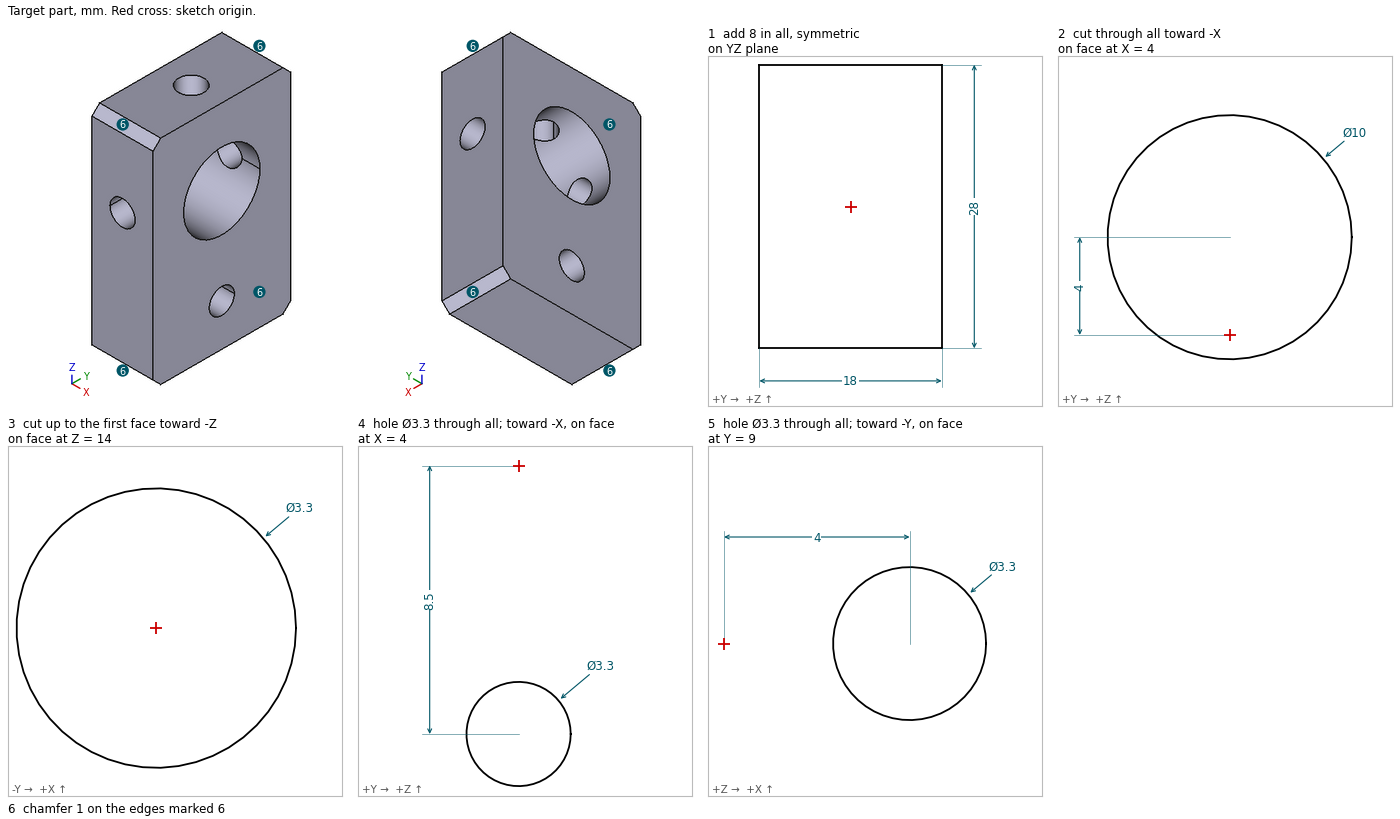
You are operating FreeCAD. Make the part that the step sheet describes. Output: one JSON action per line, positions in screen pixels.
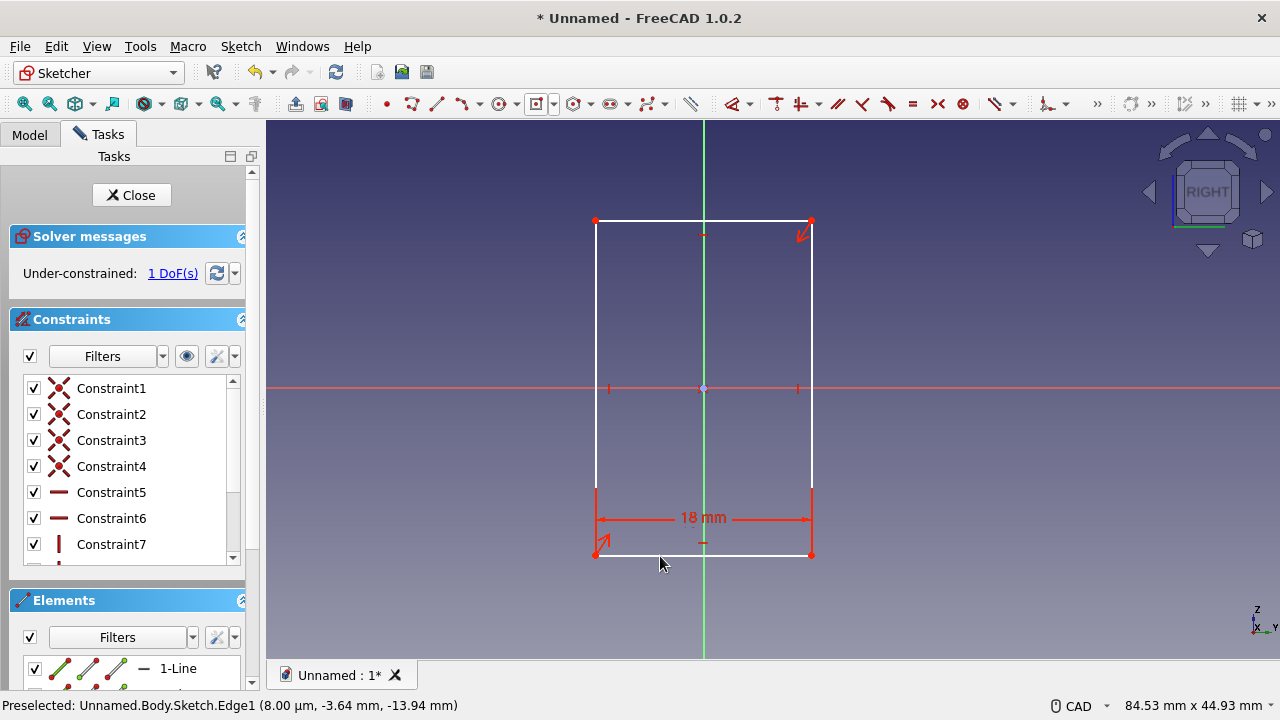
{"action": "left_click", "coordinate": [812, 455]}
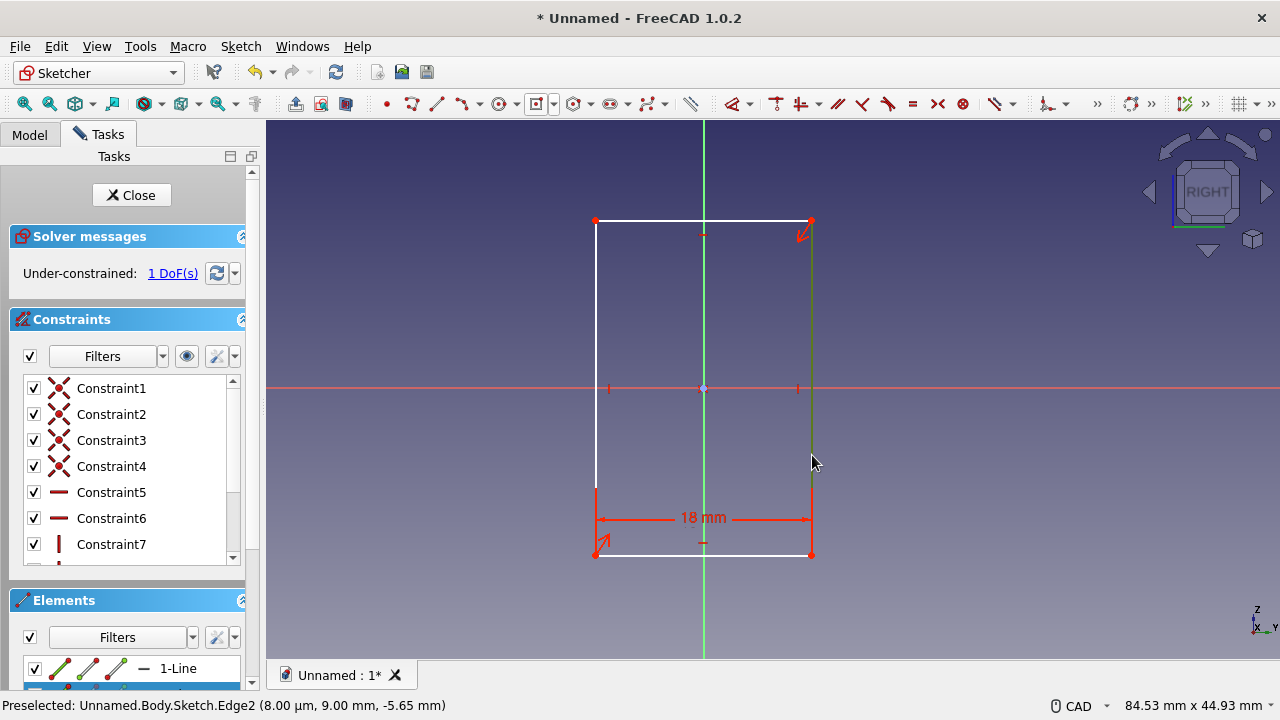
{"action": "key", "text": "i"}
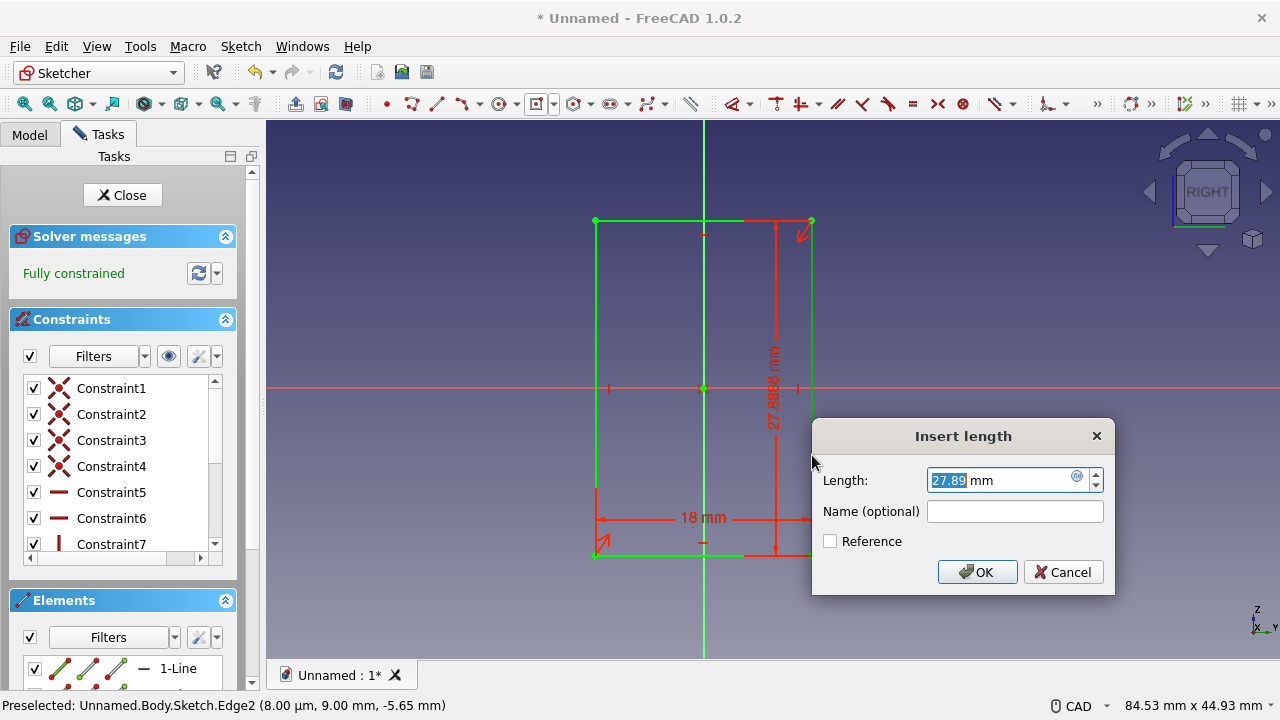
{"action": "type", "text": "28"}
{"action": "key", "text": "Return"}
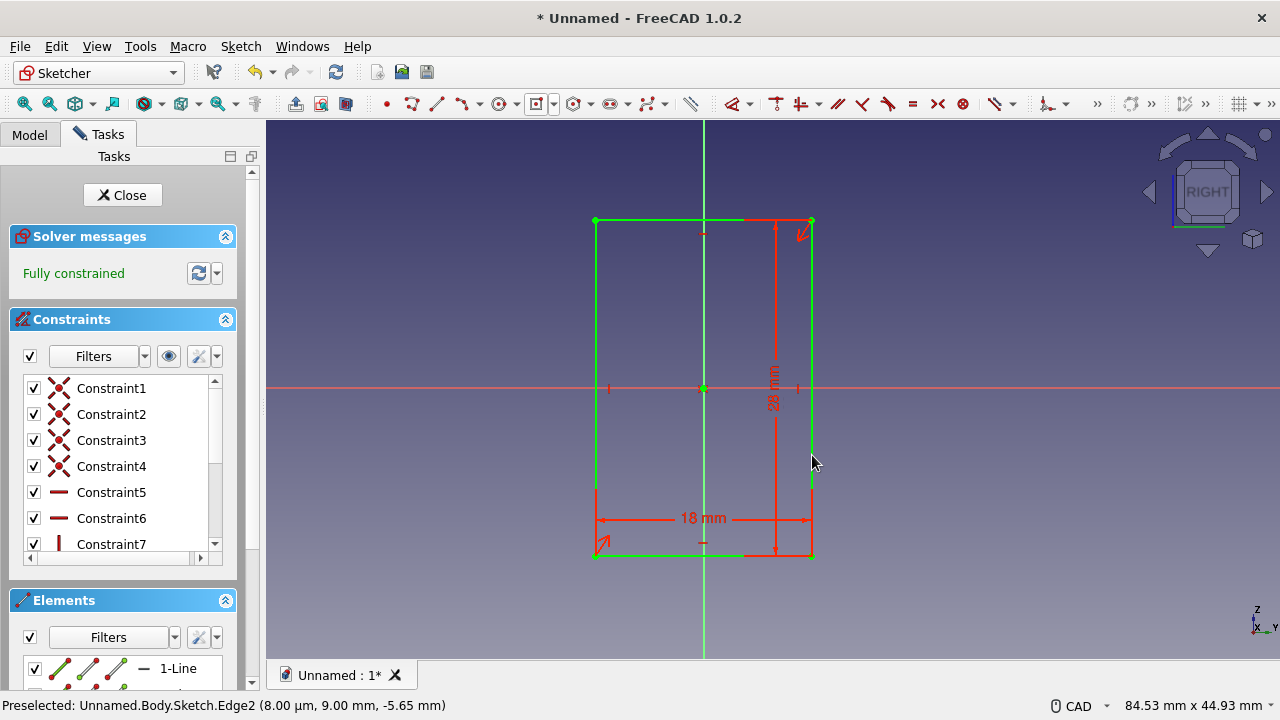
{"action": "left_click", "coordinate": [123, 195]}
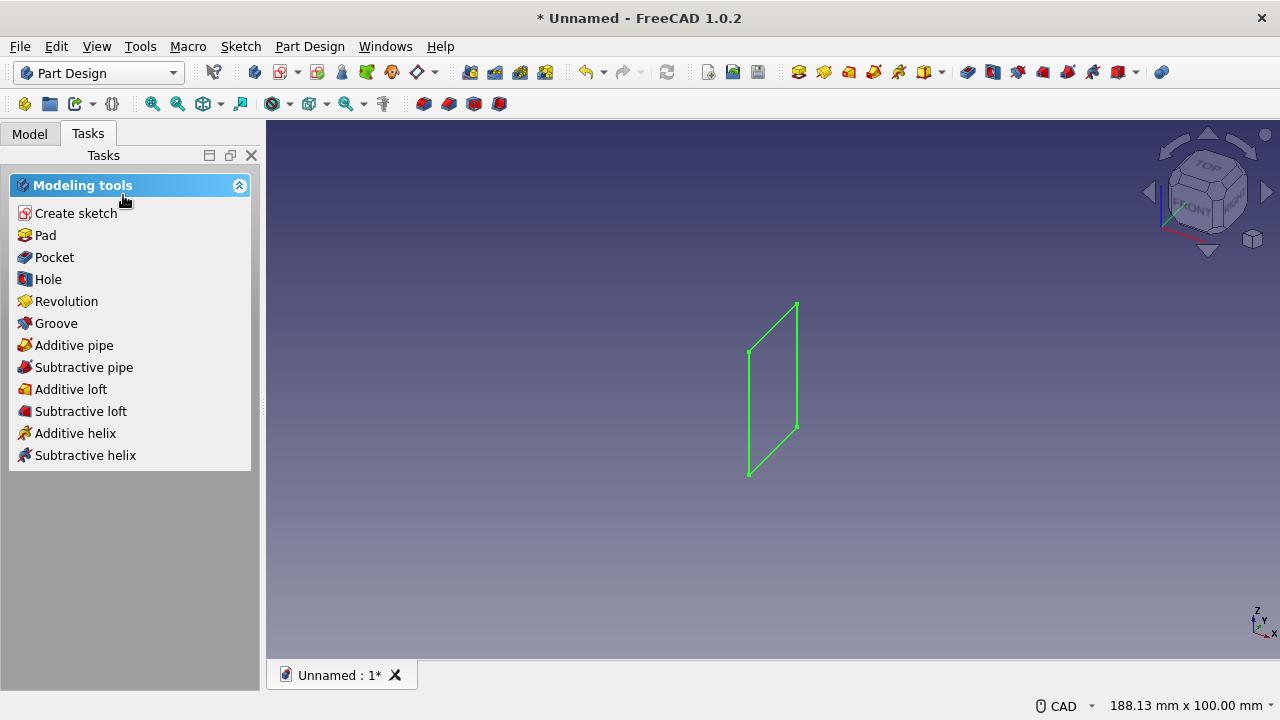
{"action": "left_click", "coordinate": [799, 72]}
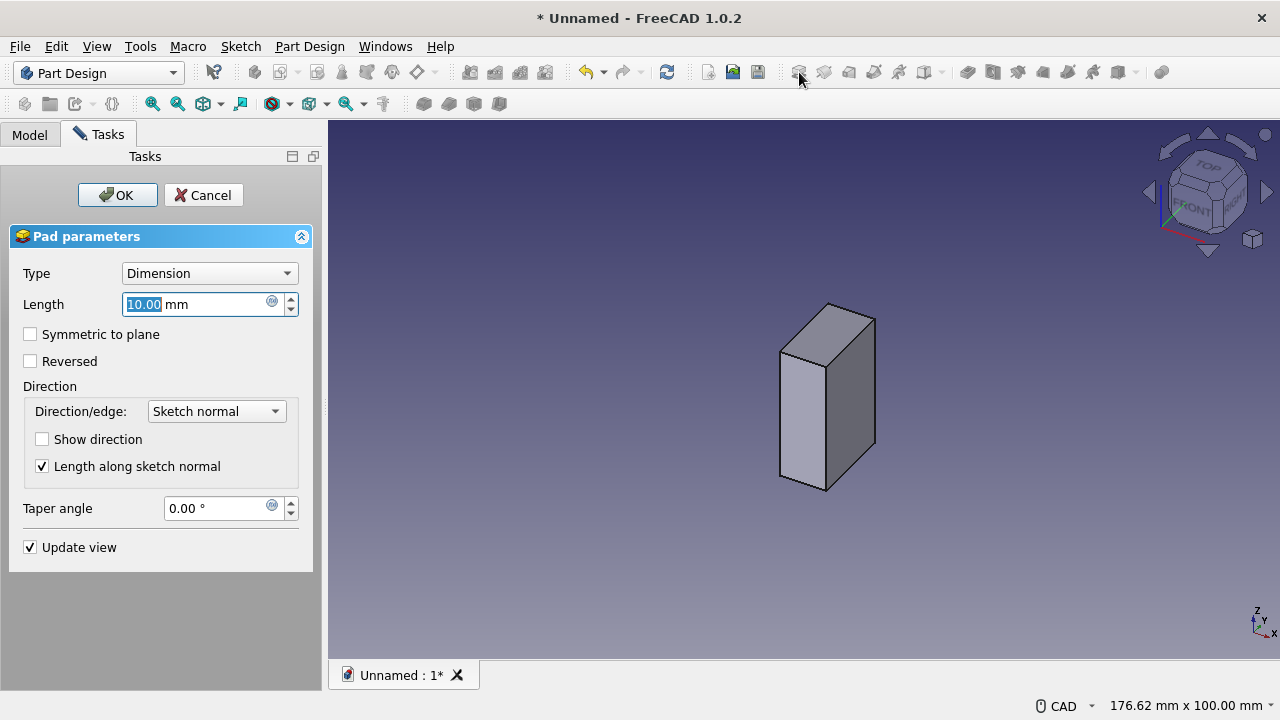
{"action": "type", "text": "8"}
{"action": "key", "text": "Tab"}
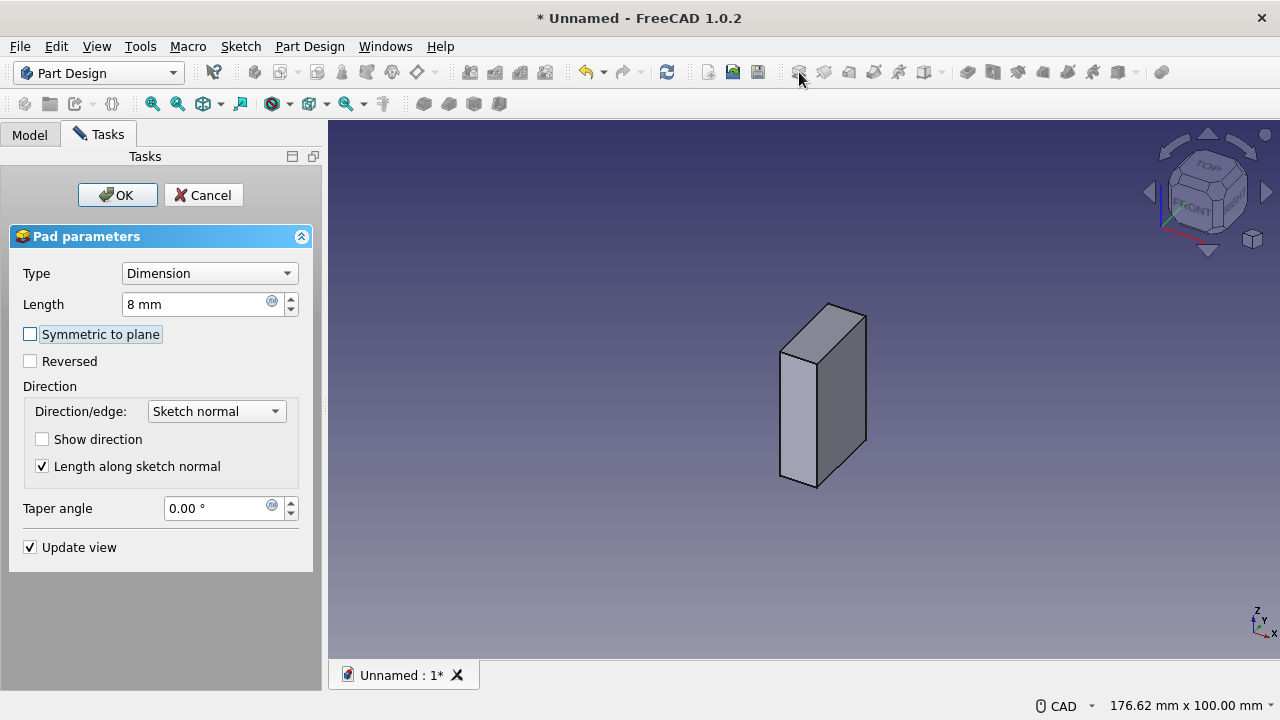
{"action": "left_click", "coordinate": [31, 334]}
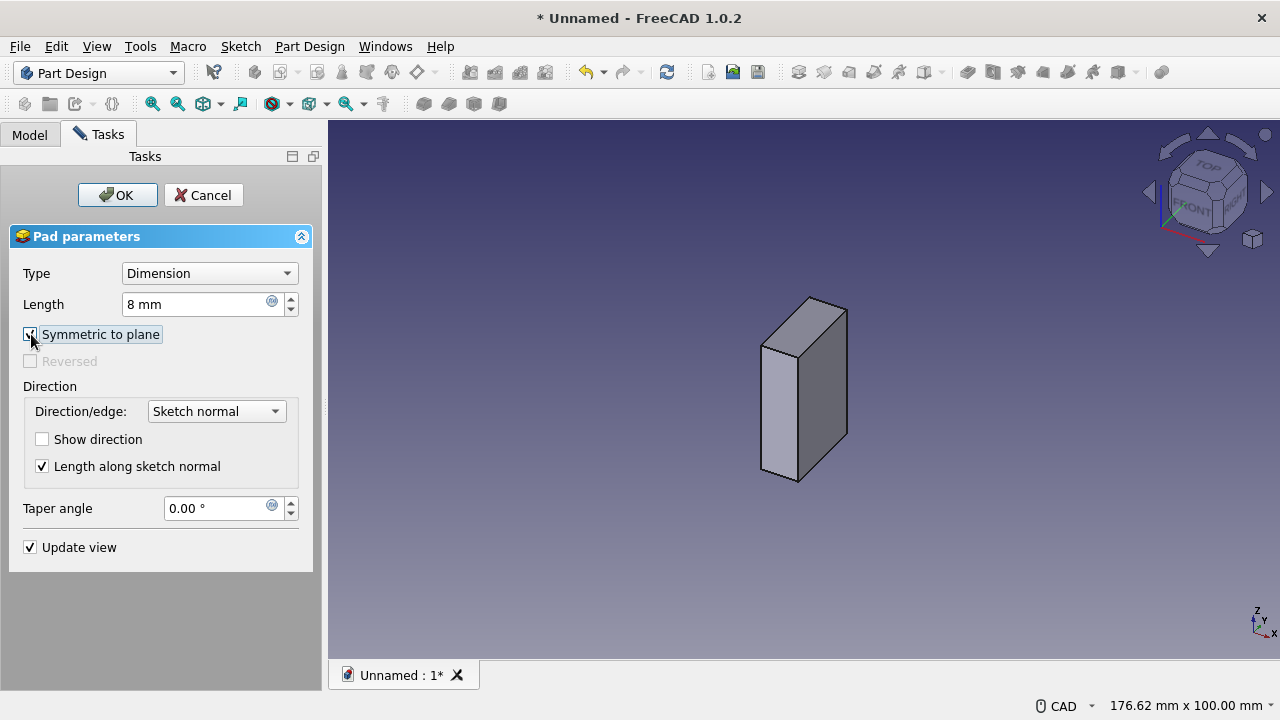
{"action": "left_click", "coordinate": [118, 195]}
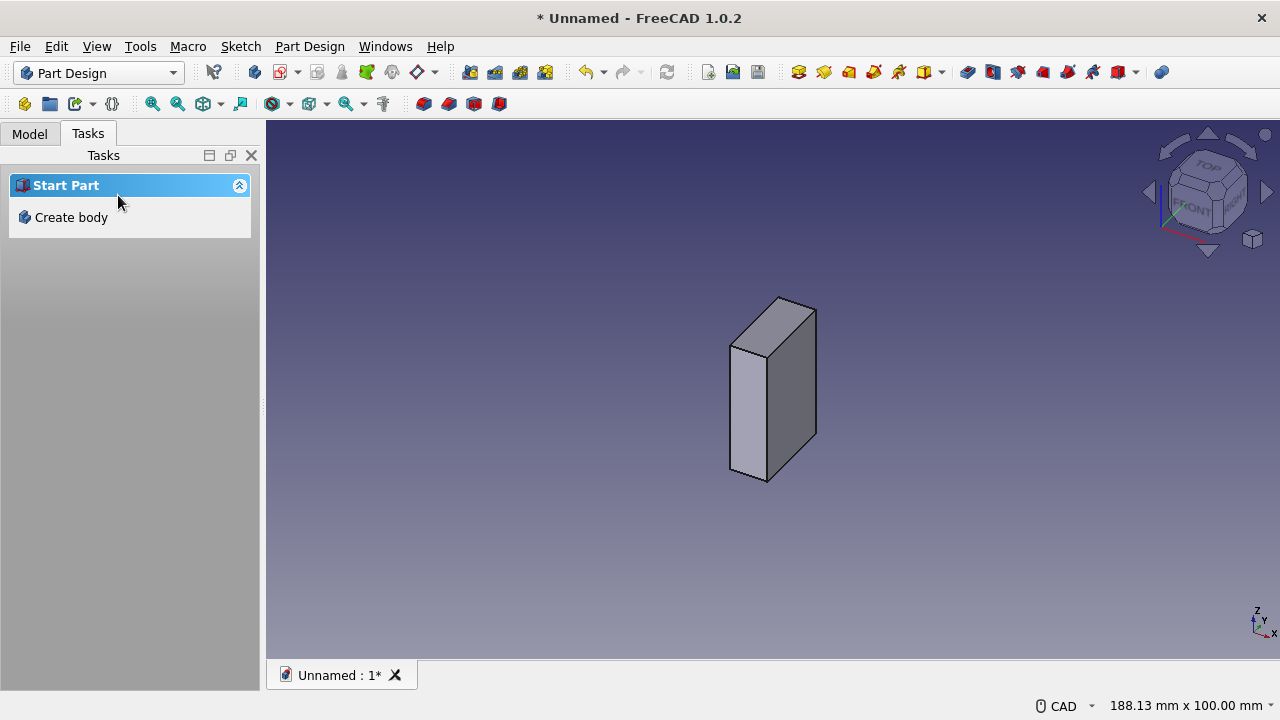
{"action": "left_click", "coordinate": [153, 104]}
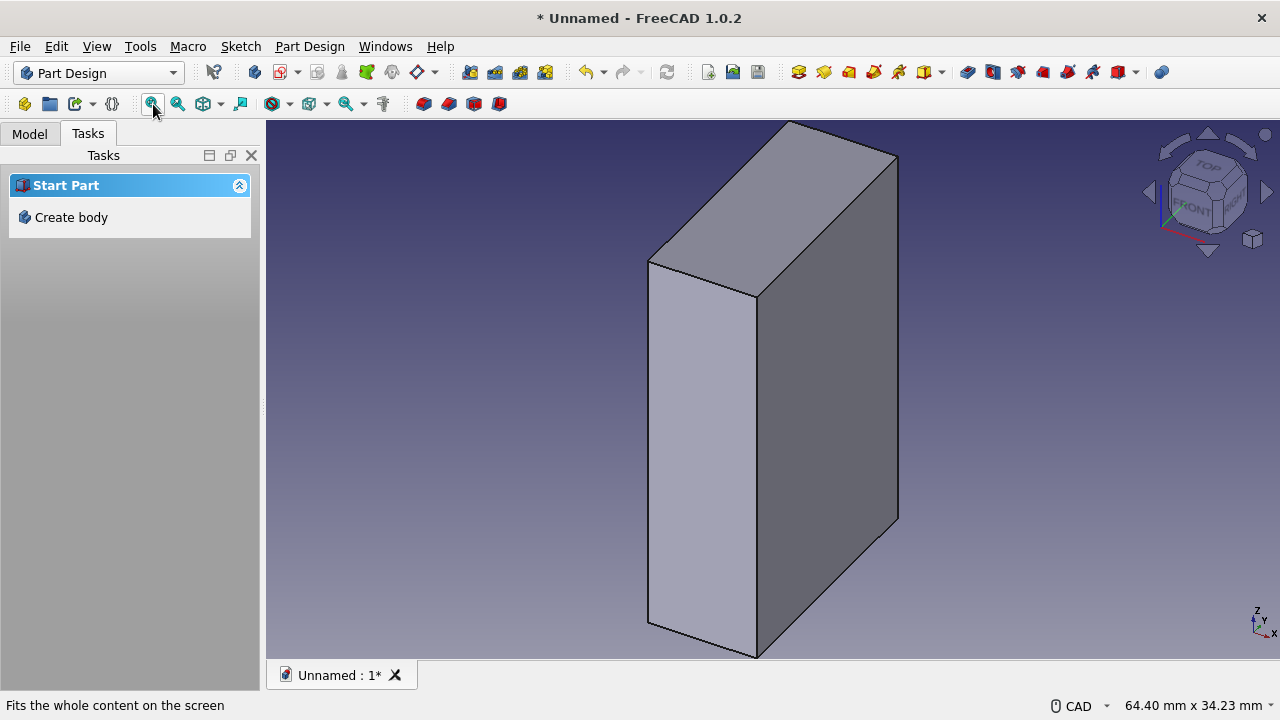
{"action": "left_click", "coordinate": [828, 407]}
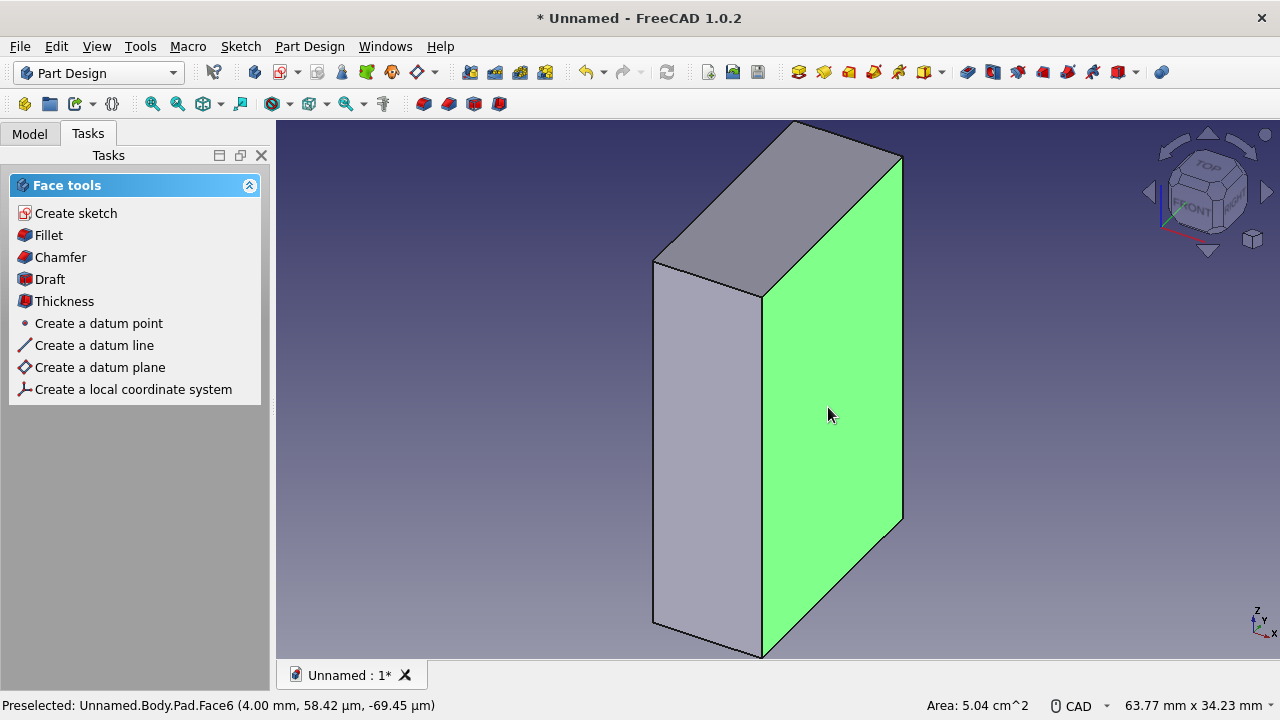
{"action": "left_click", "coordinate": [280, 72]}